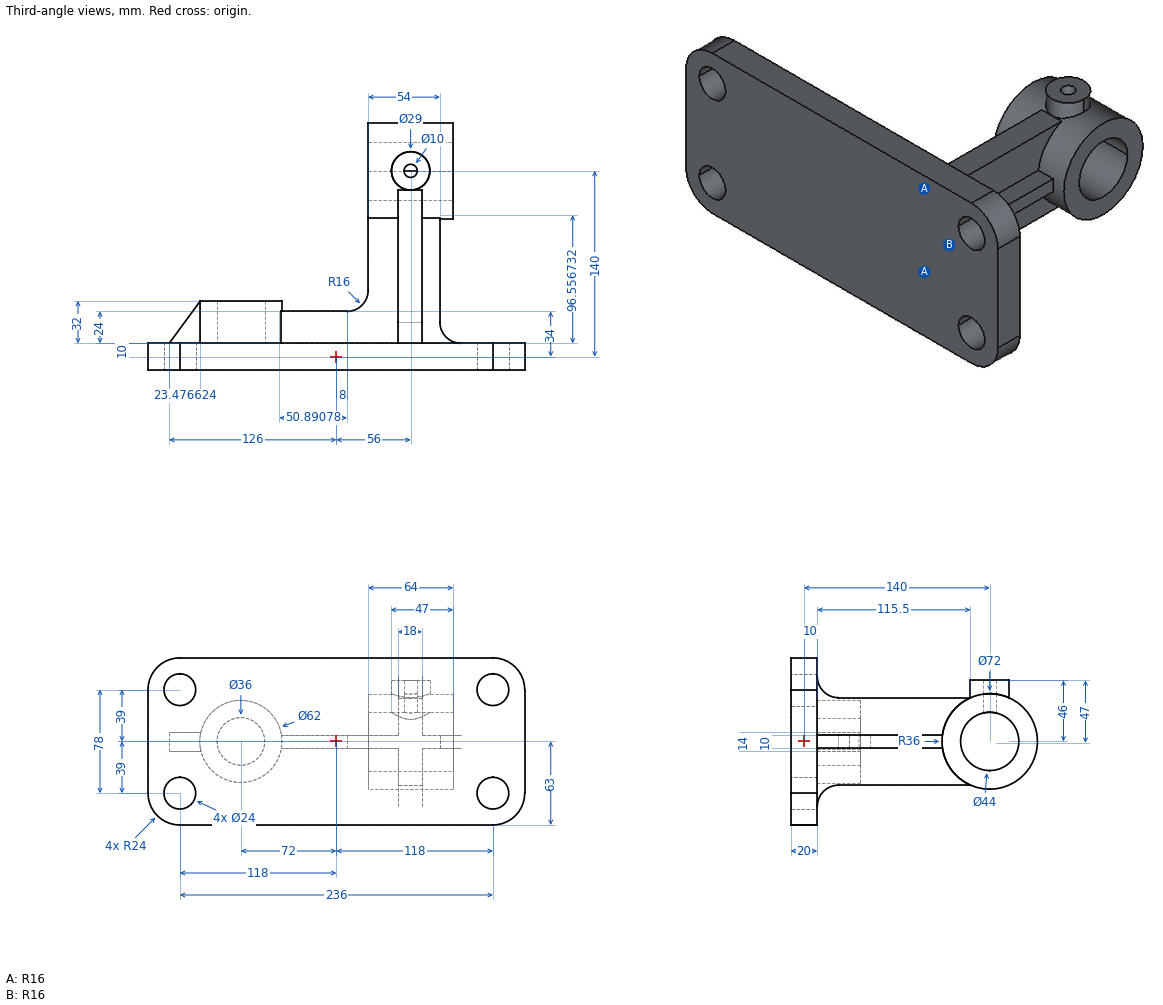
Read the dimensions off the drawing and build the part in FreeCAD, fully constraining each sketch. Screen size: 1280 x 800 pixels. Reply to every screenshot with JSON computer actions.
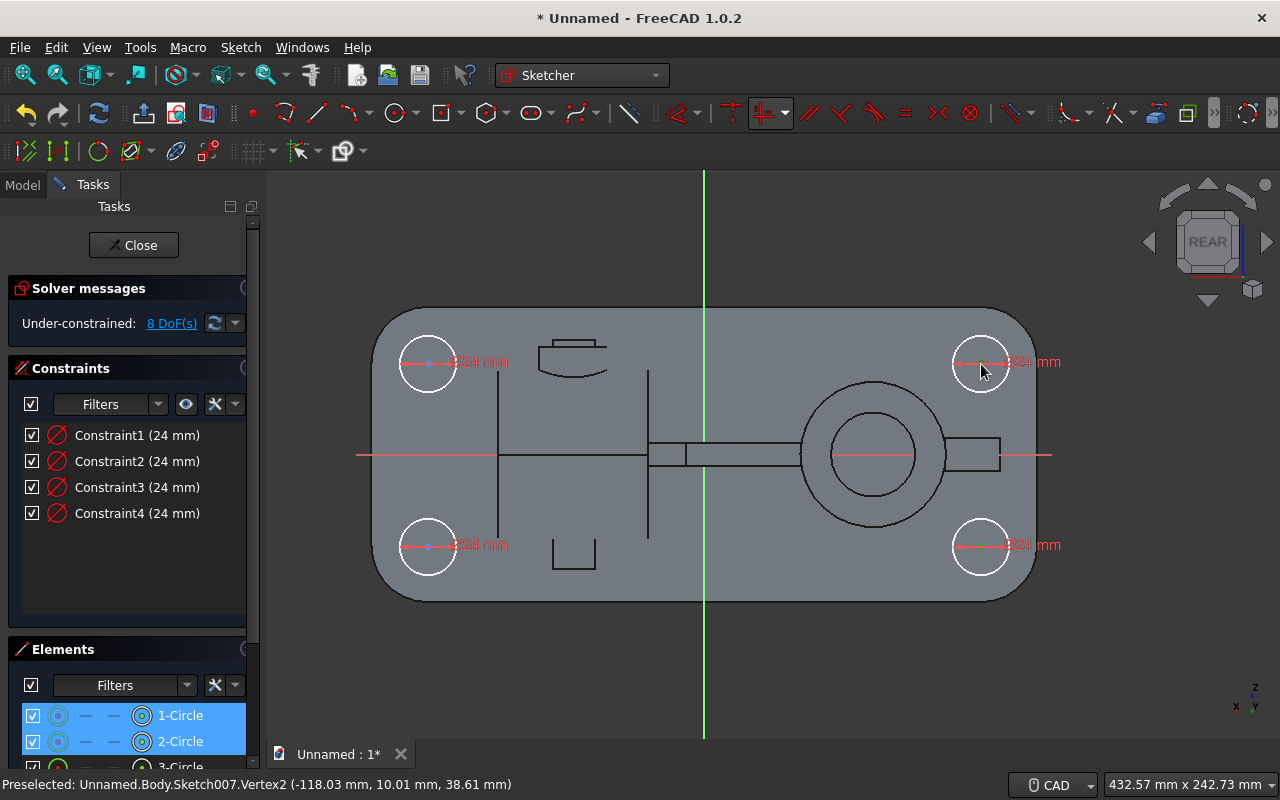
{"action": "left_click", "coordinate": [788, 114]}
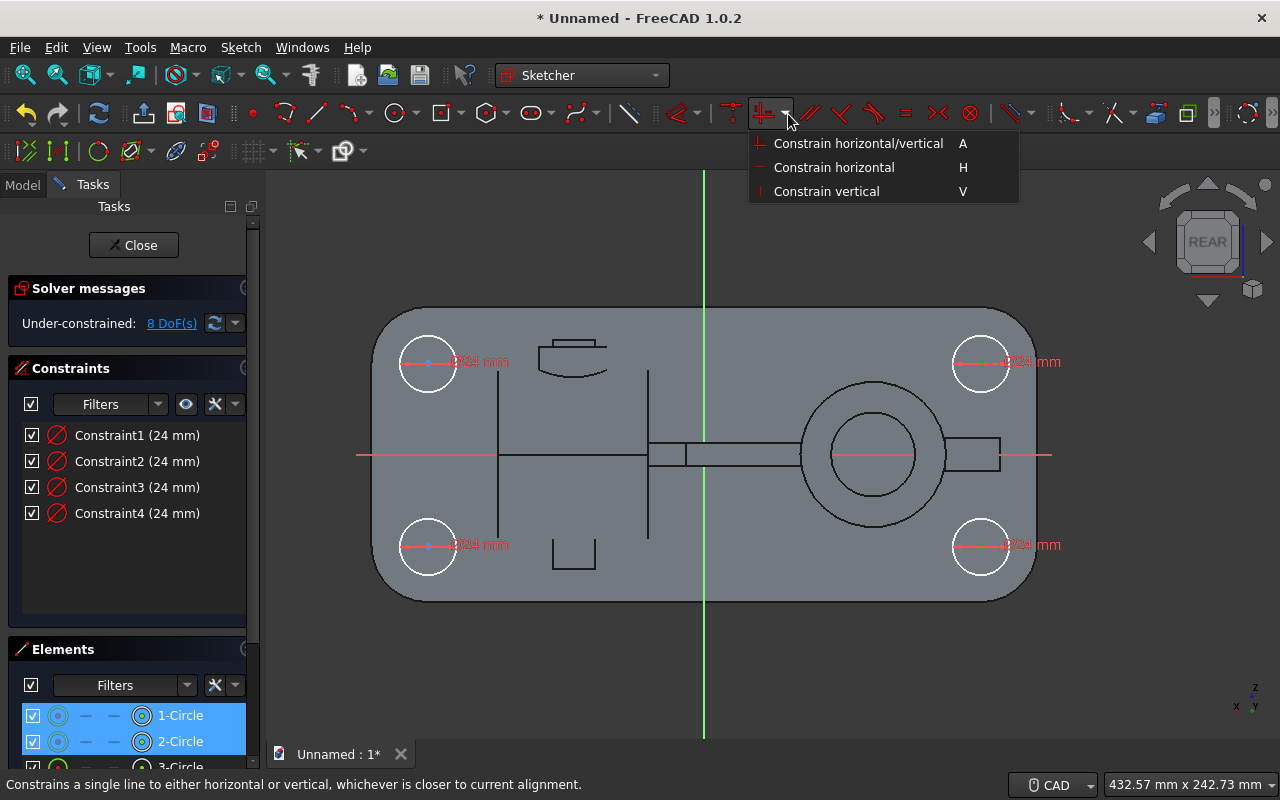
{"action": "left_click", "coordinate": [884, 191]}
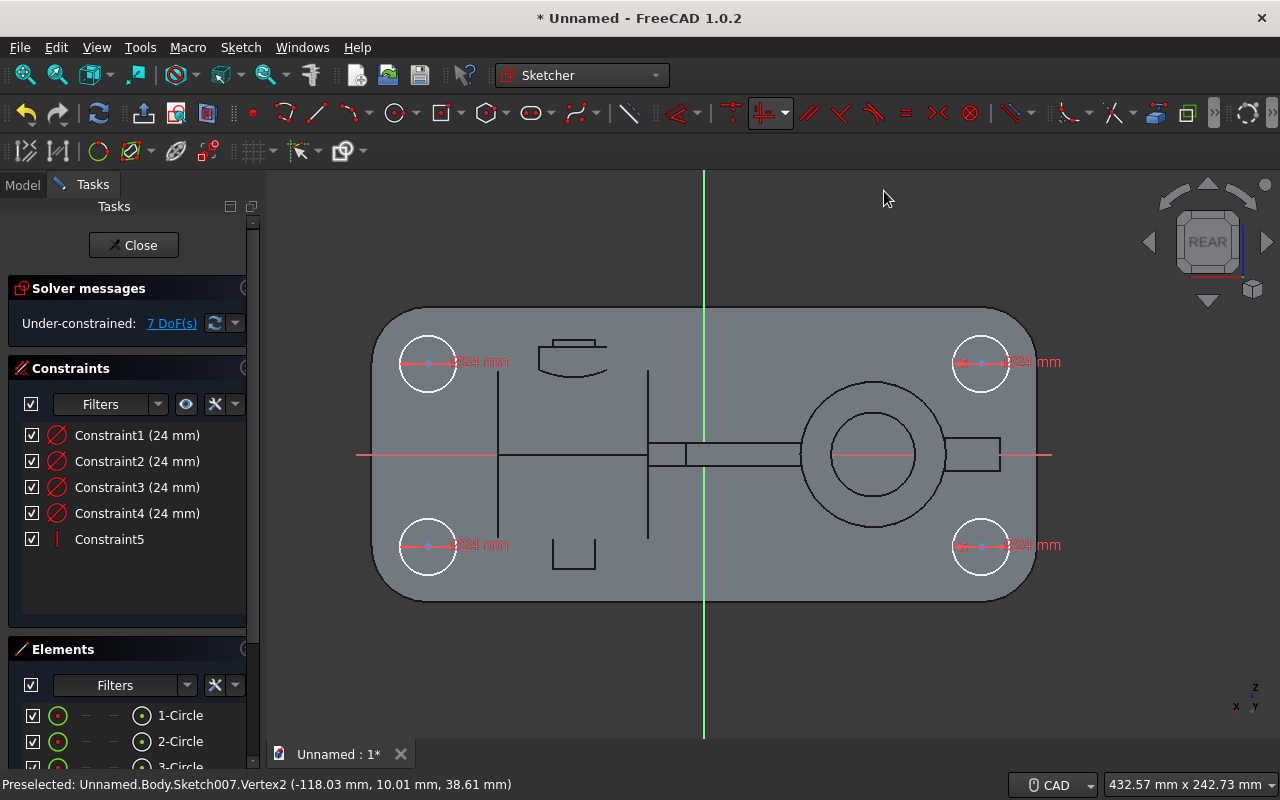
{"action": "left_click", "coordinate": [981, 364]}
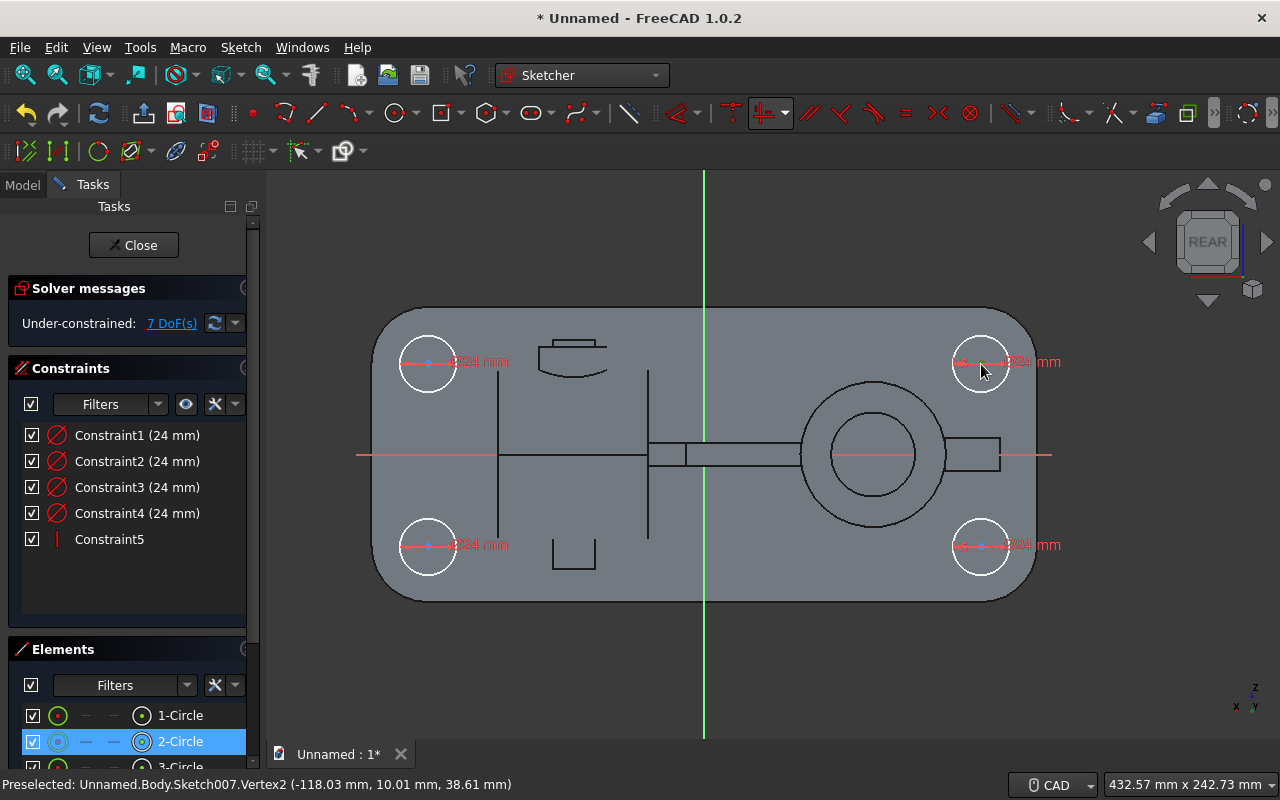
{"action": "left_click", "coordinate": [428, 364]}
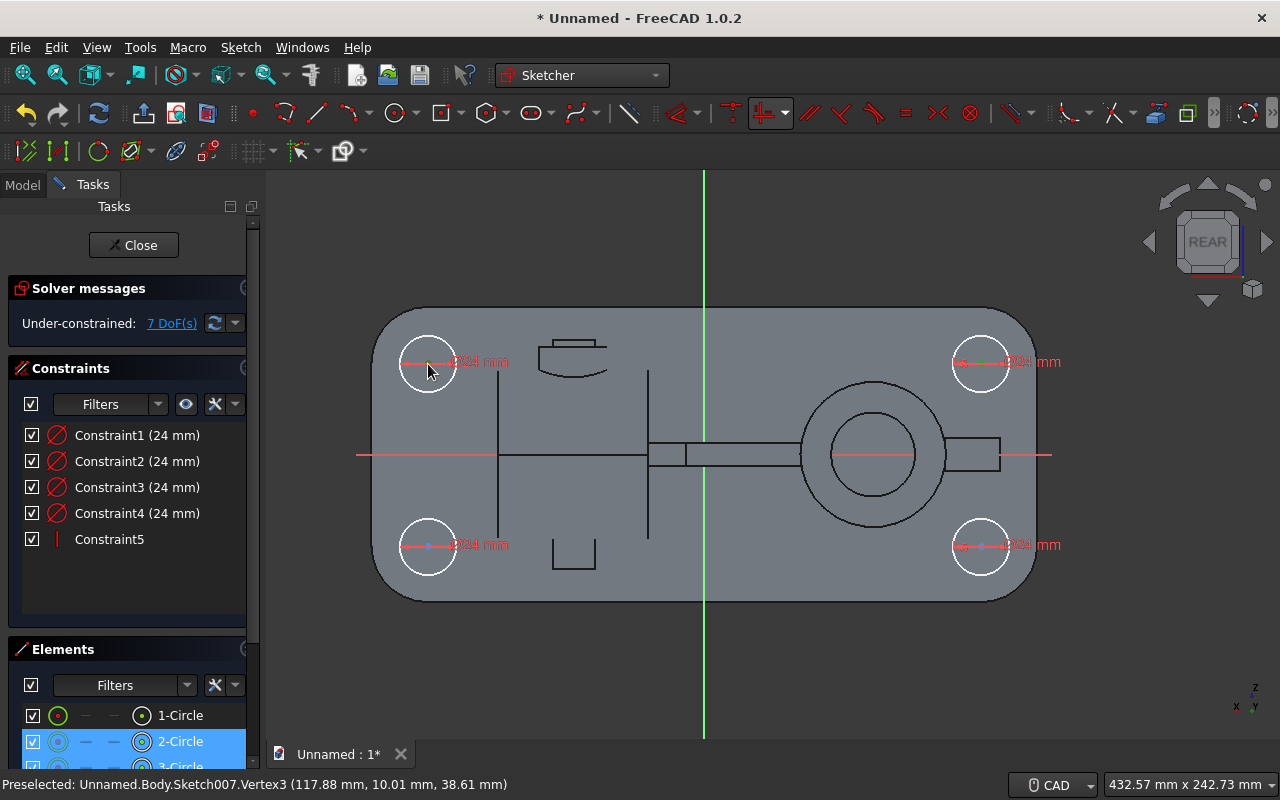
{"action": "key", "text": "h"}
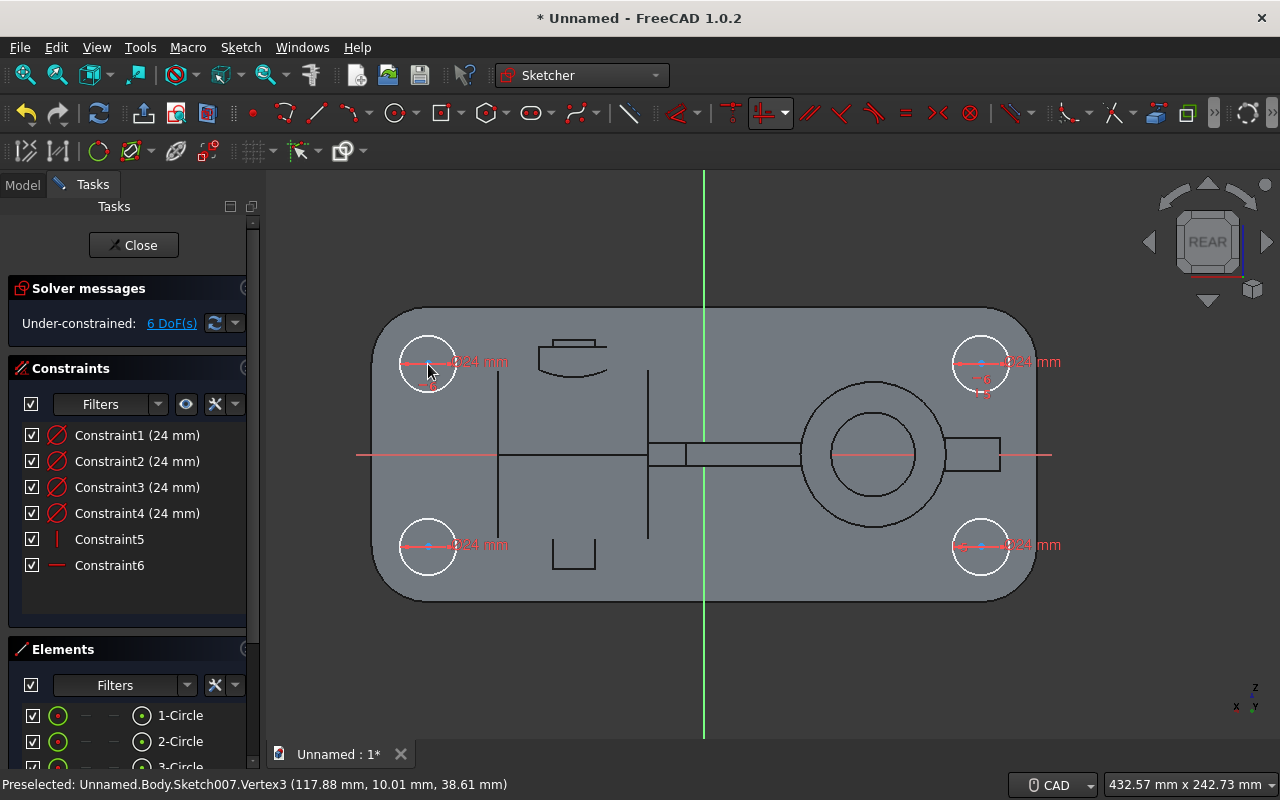
{"action": "left_click", "coordinate": [428, 364]}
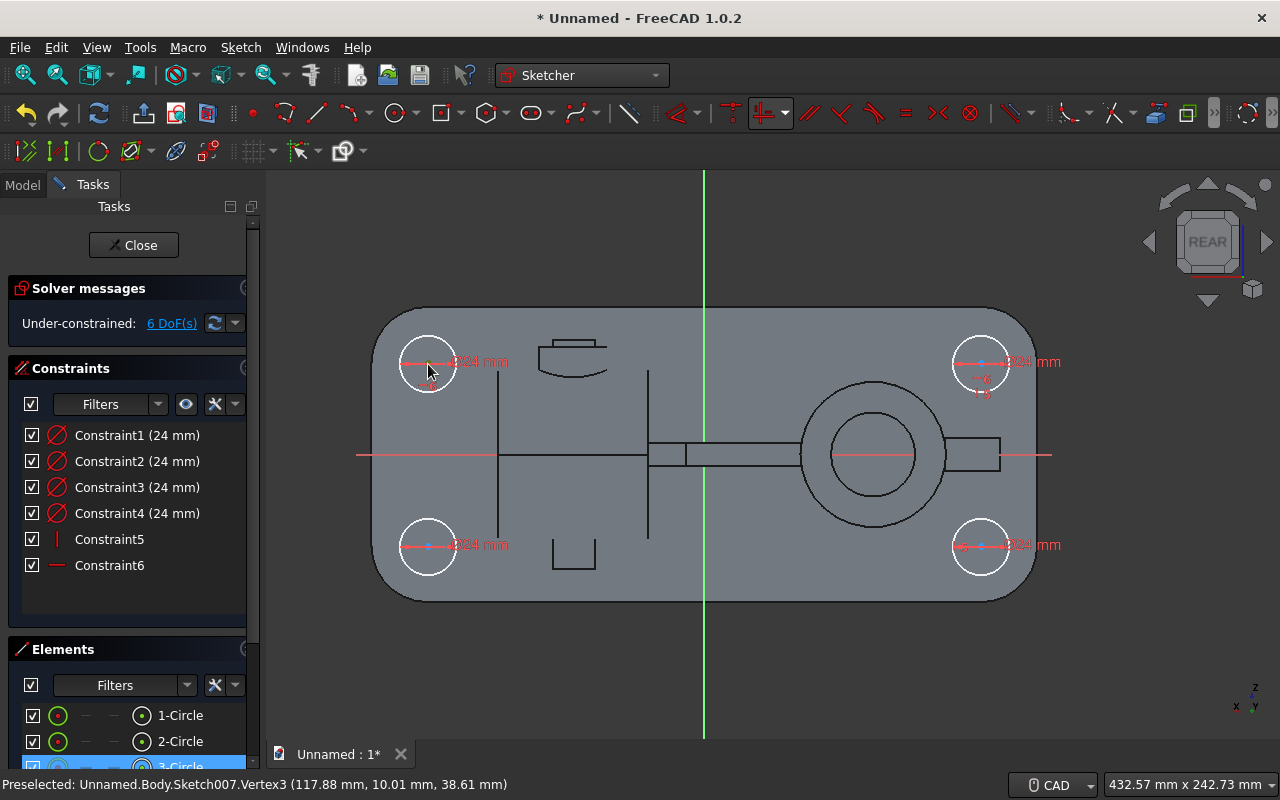
{"action": "left_click", "coordinate": [428, 547]}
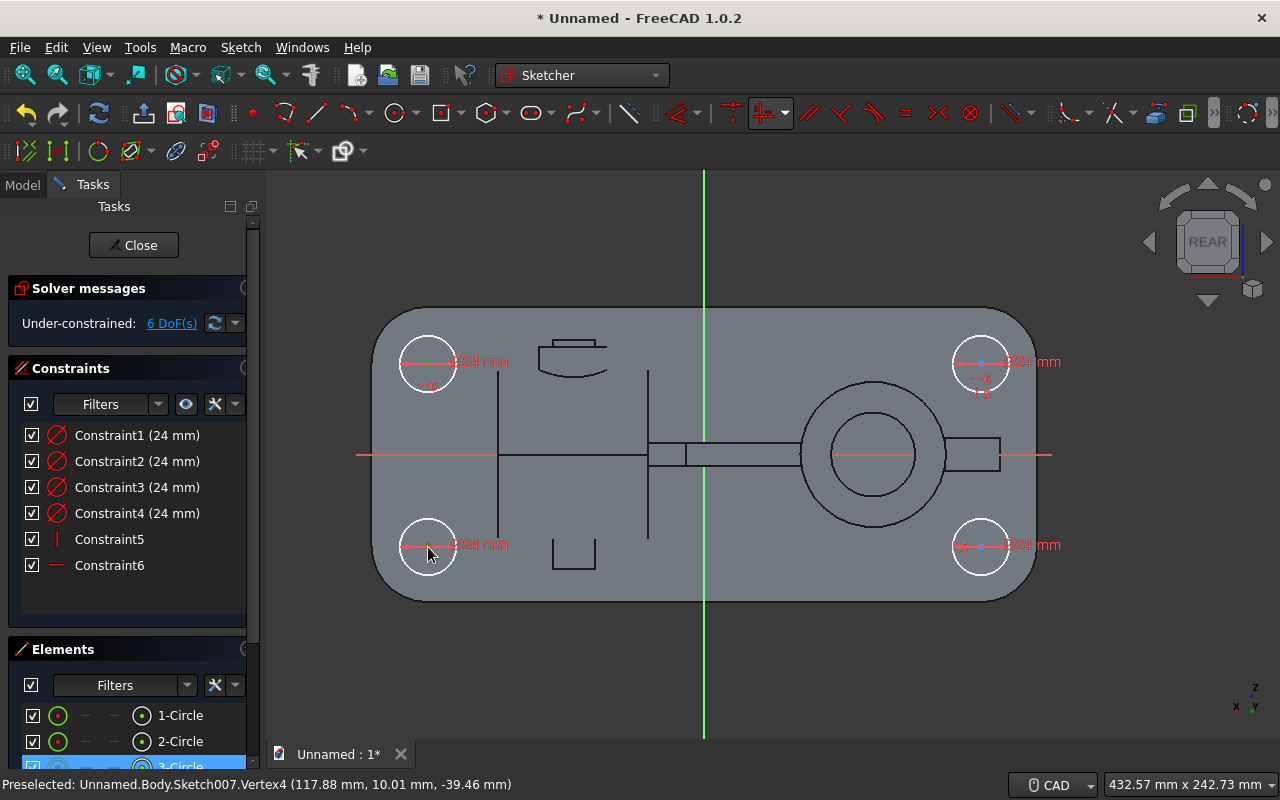
{"action": "key", "text": "v"}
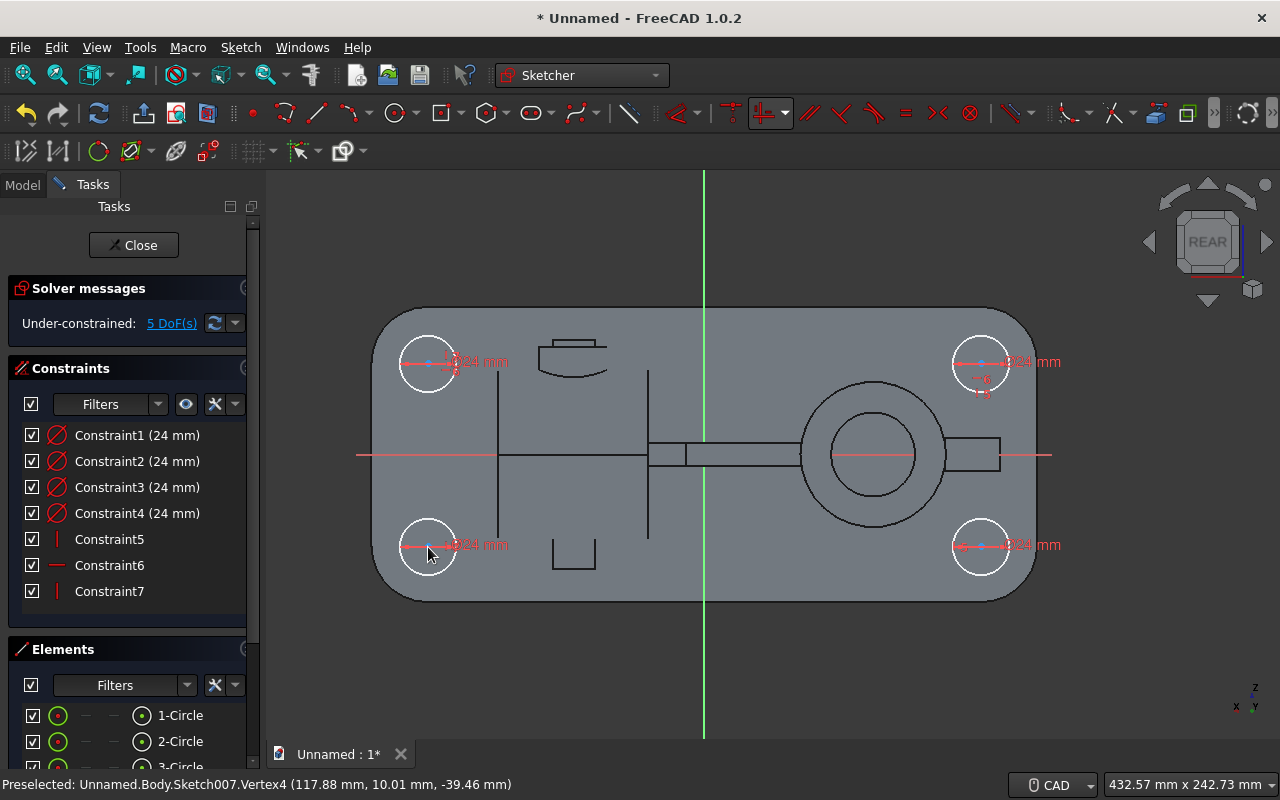
{"action": "left_click", "coordinate": [981, 547]}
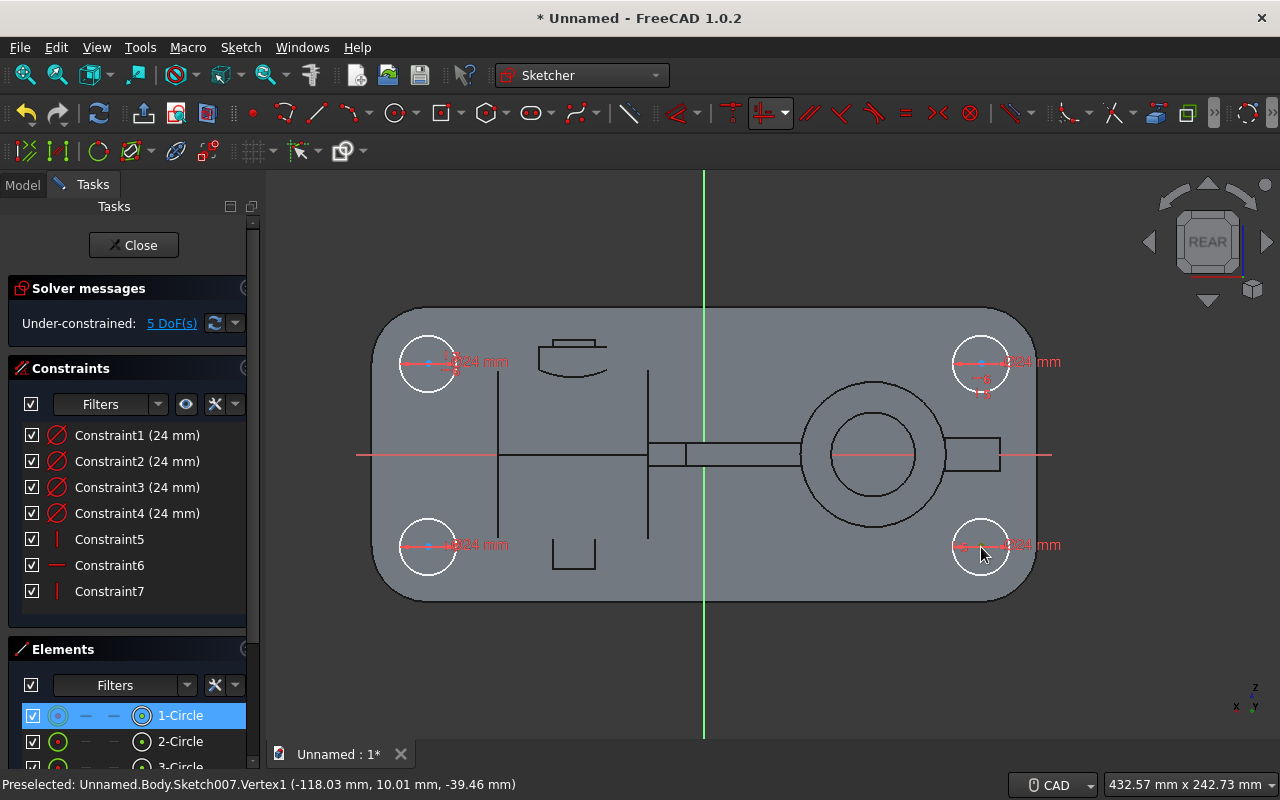
{"action": "left_click", "coordinate": [428, 547]}